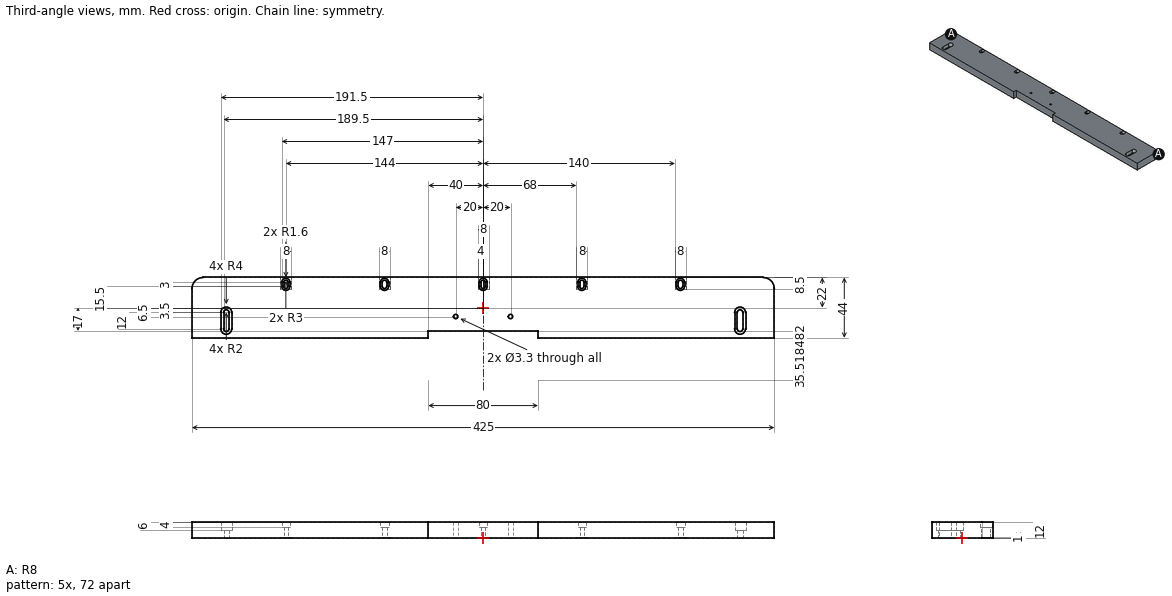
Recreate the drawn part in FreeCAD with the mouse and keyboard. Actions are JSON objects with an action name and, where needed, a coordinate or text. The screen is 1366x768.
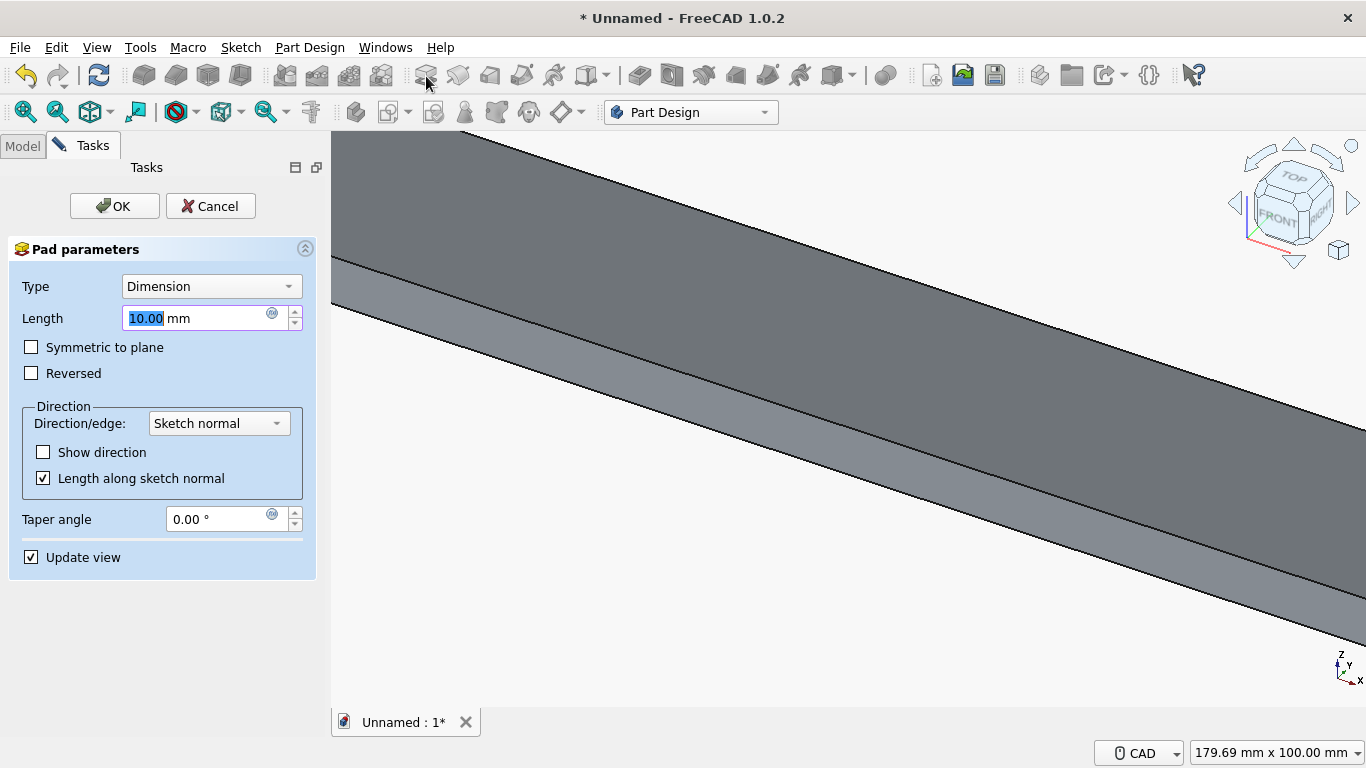
{"action": "type", "text": "12"}
{"action": "key", "text": "Tab"}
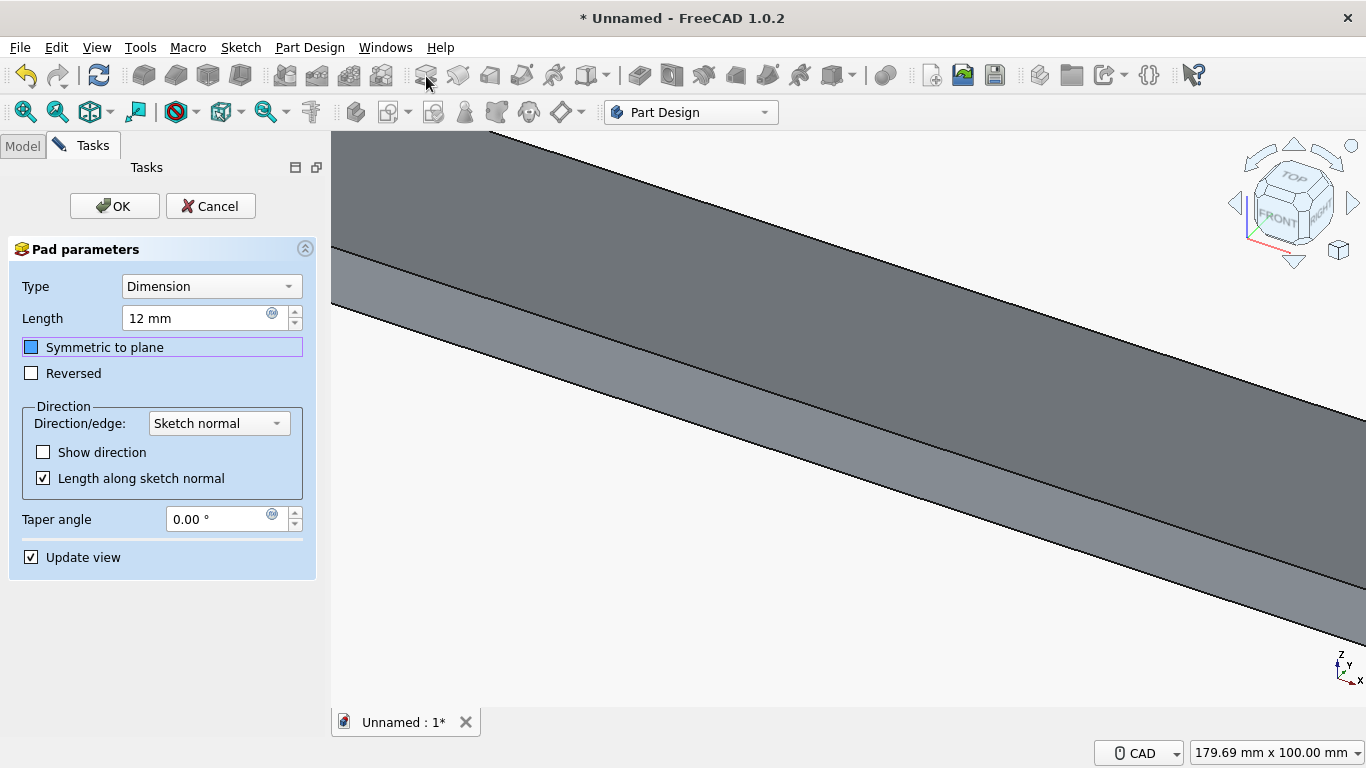
{"action": "left_click", "coordinate": [115, 206]}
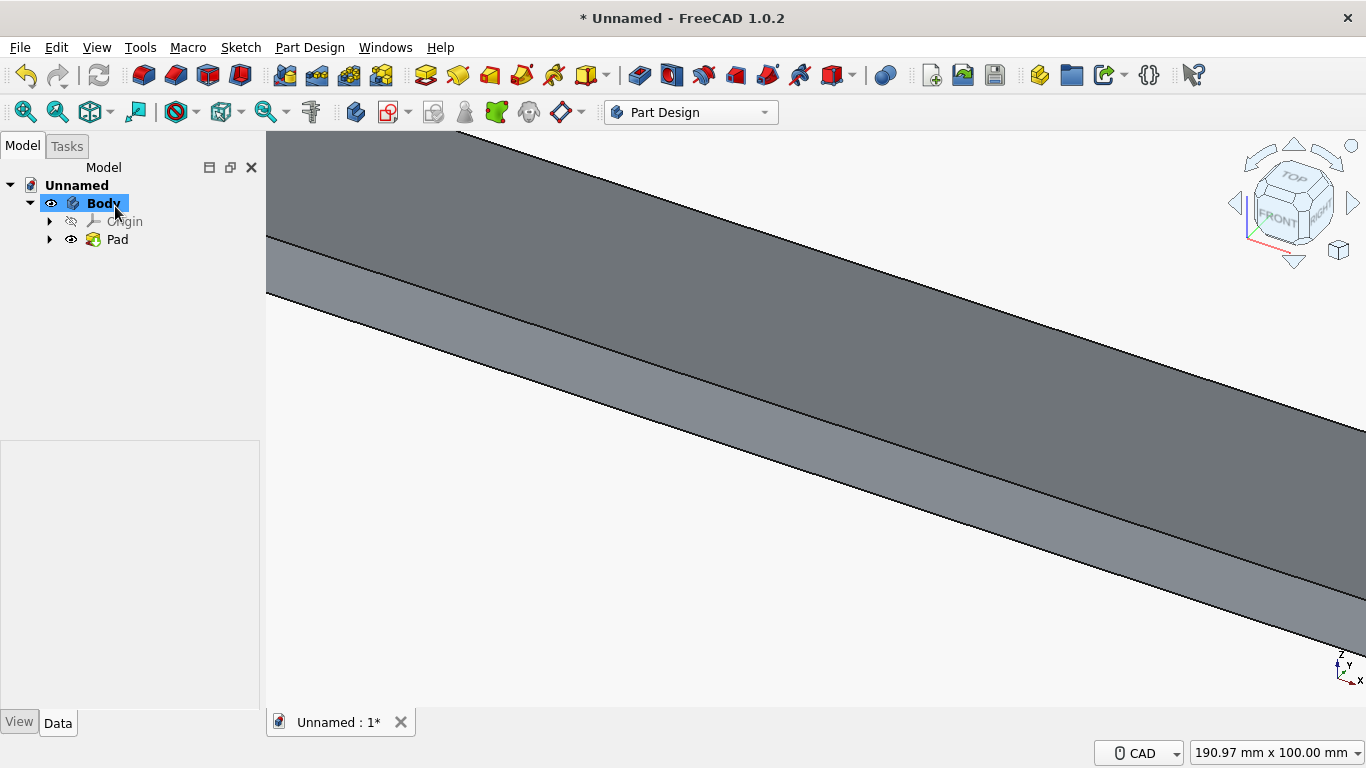
{"action": "left_click", "coordinate": [26, 112]}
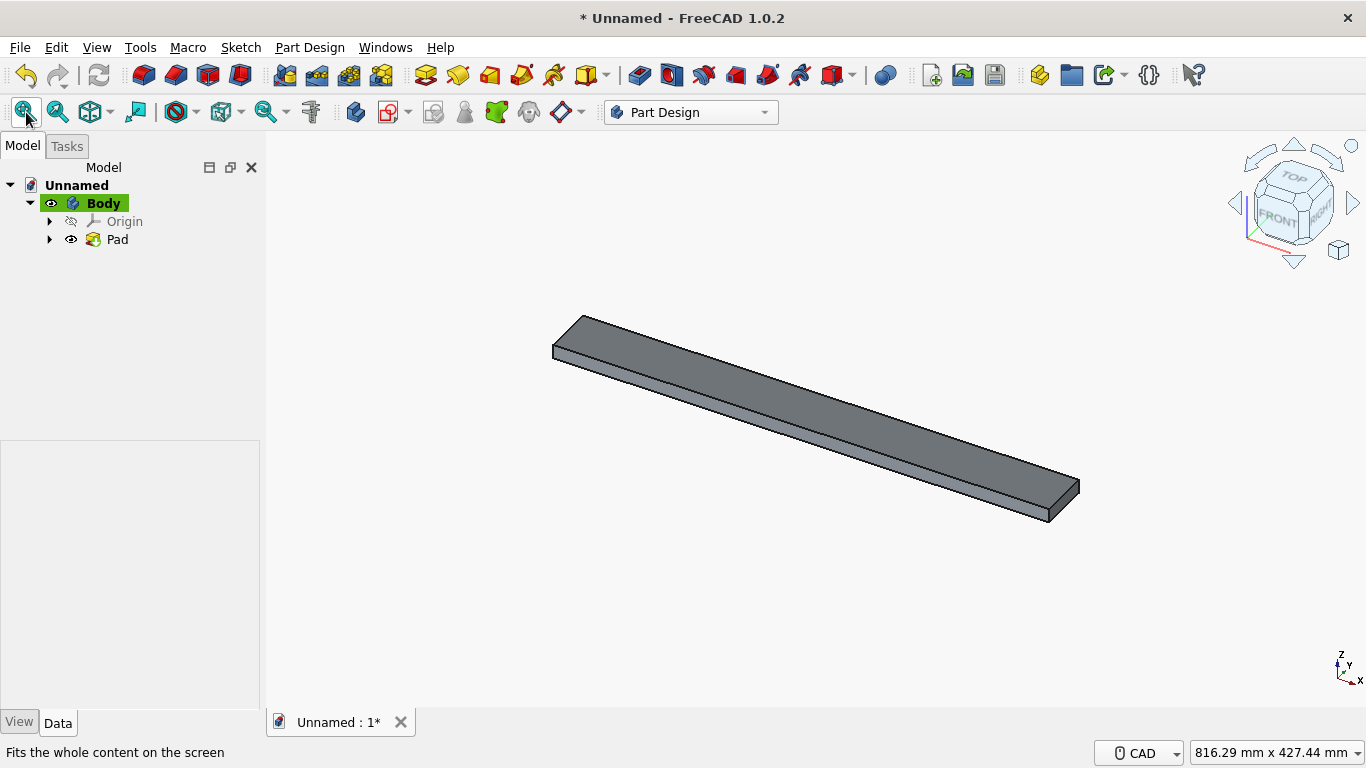
{"action": "scroll", "coordinate": [583, 321], "scroll_direction": "up", "scroll_amount": 5}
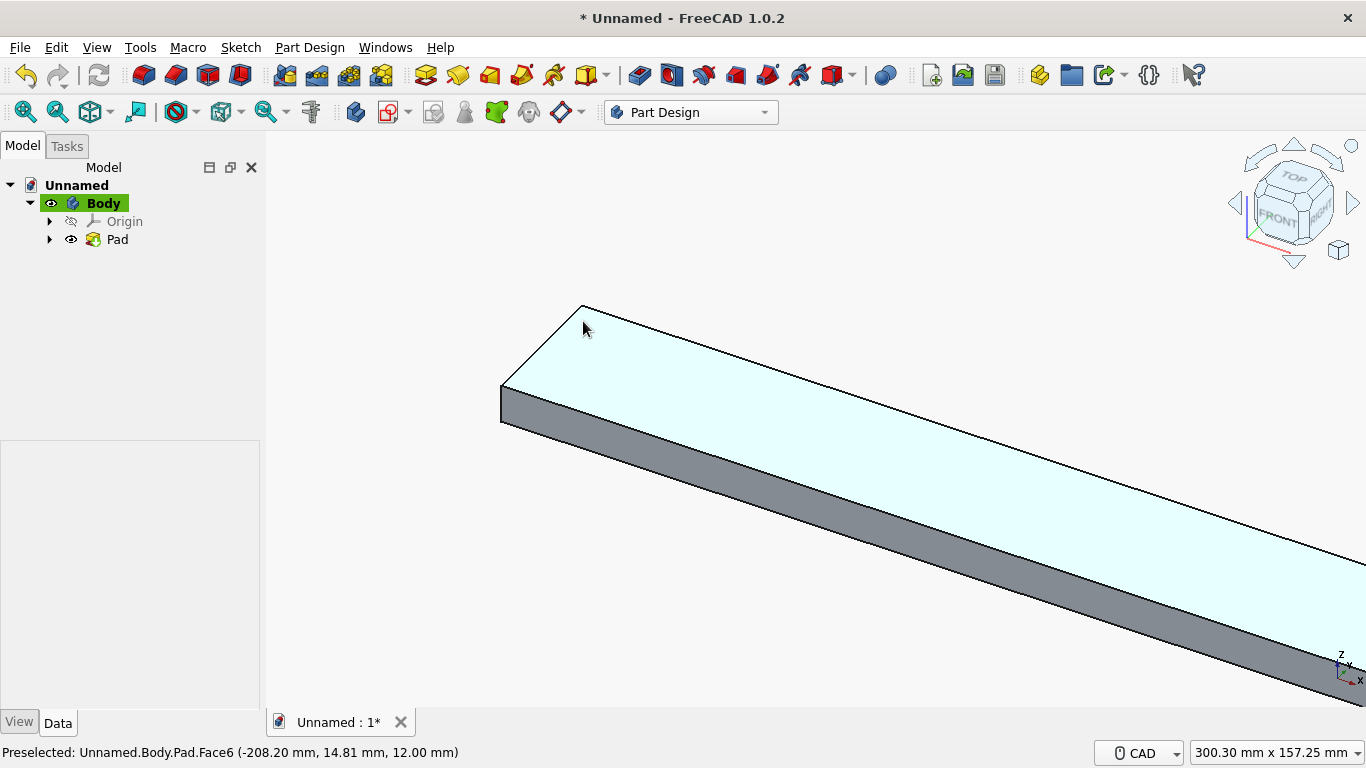
{"action": "key", "text": "v f"}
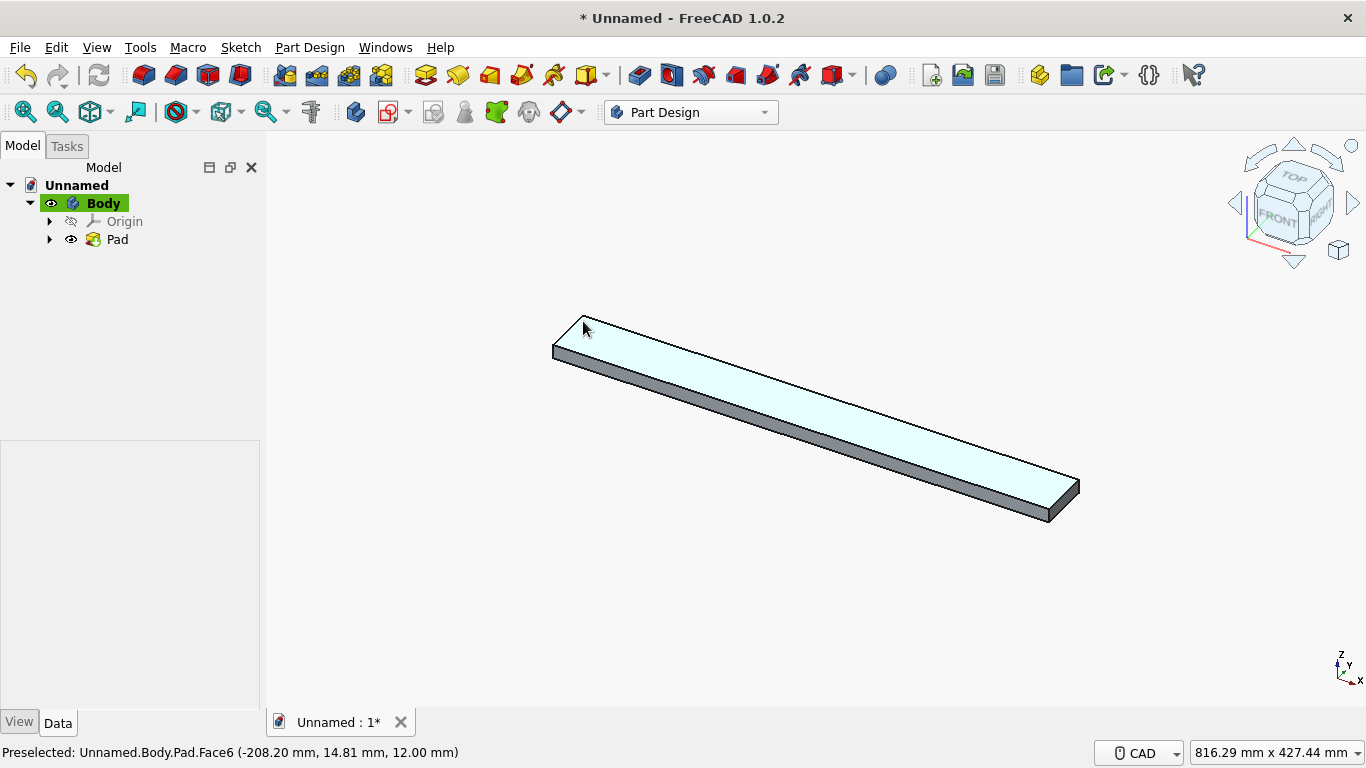
{"action": "key", "text": "0"}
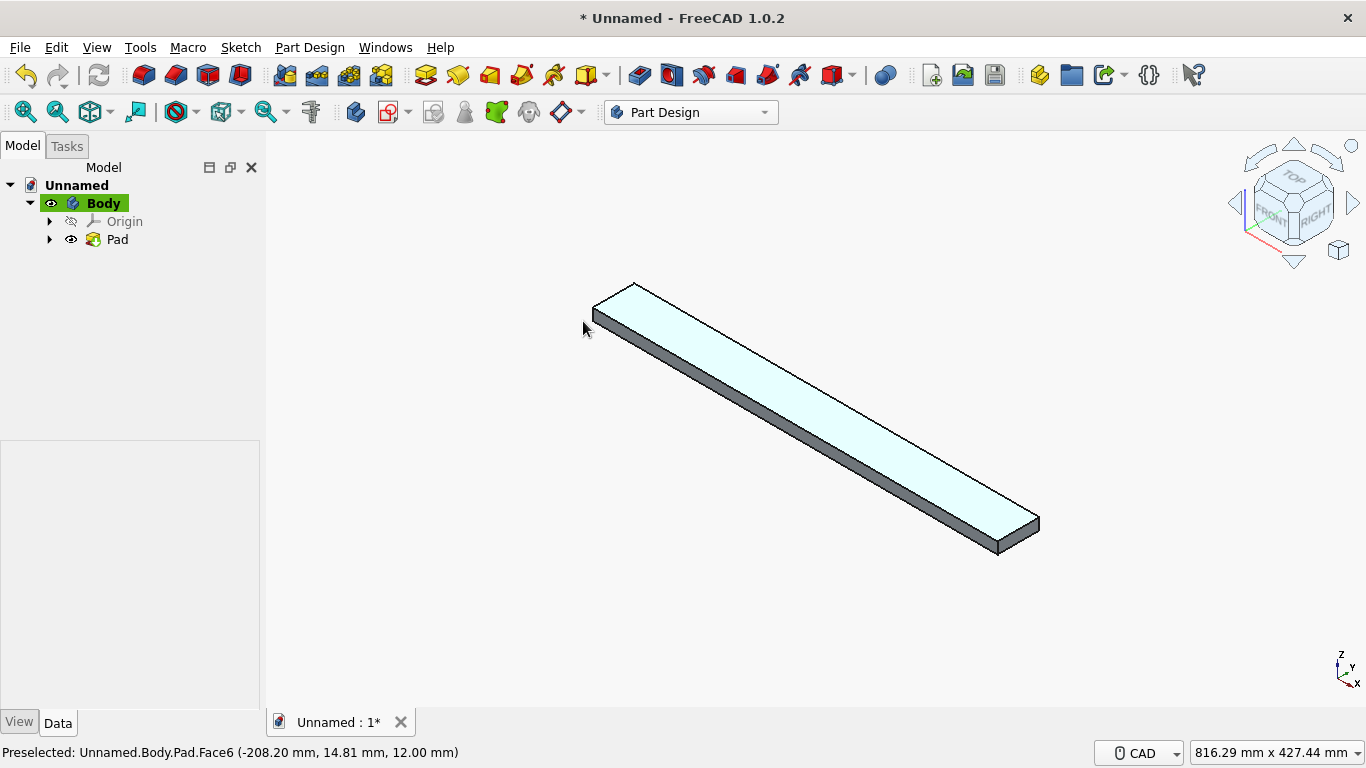
{"action": "scroll", "coordinate": [634, 289], "scroll_direction": "up", "scroll_amount": 5}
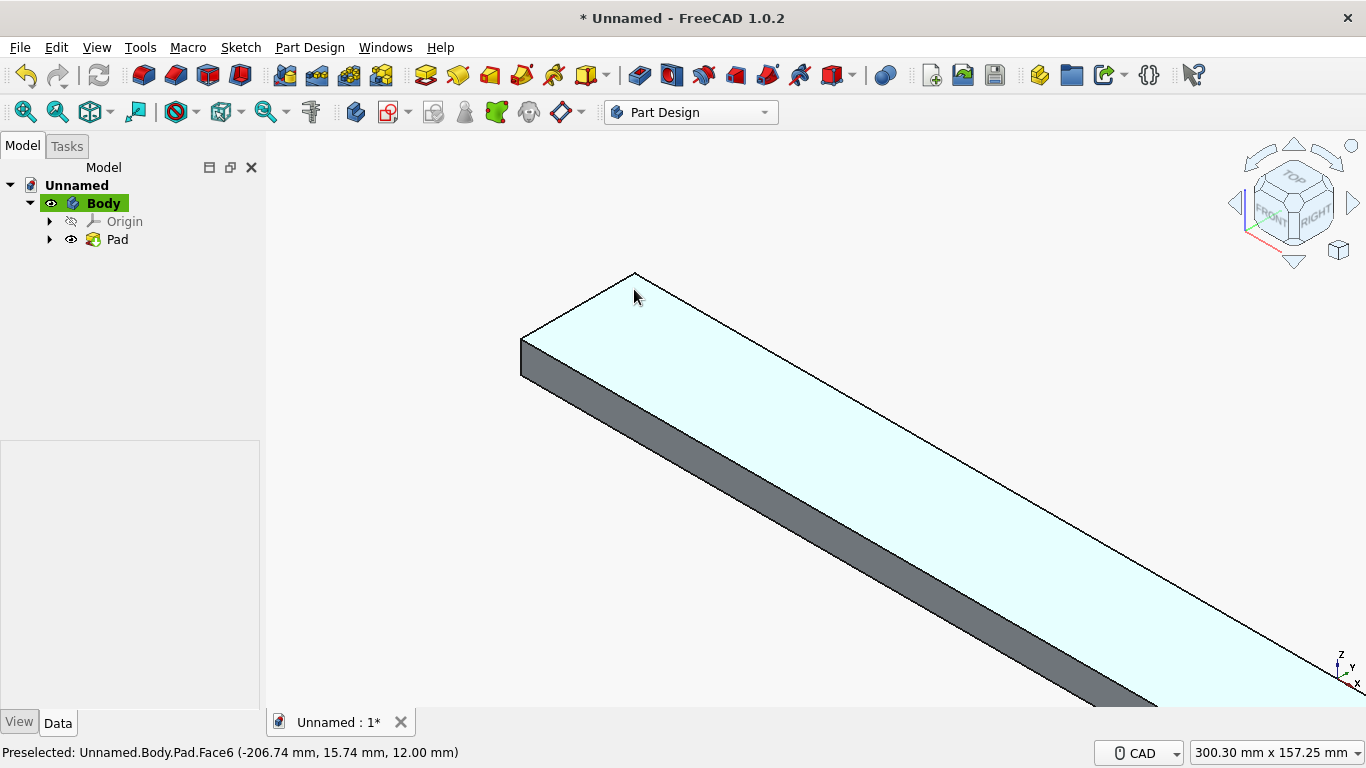
{"action": "left_click", "coordinate": [26, 112]}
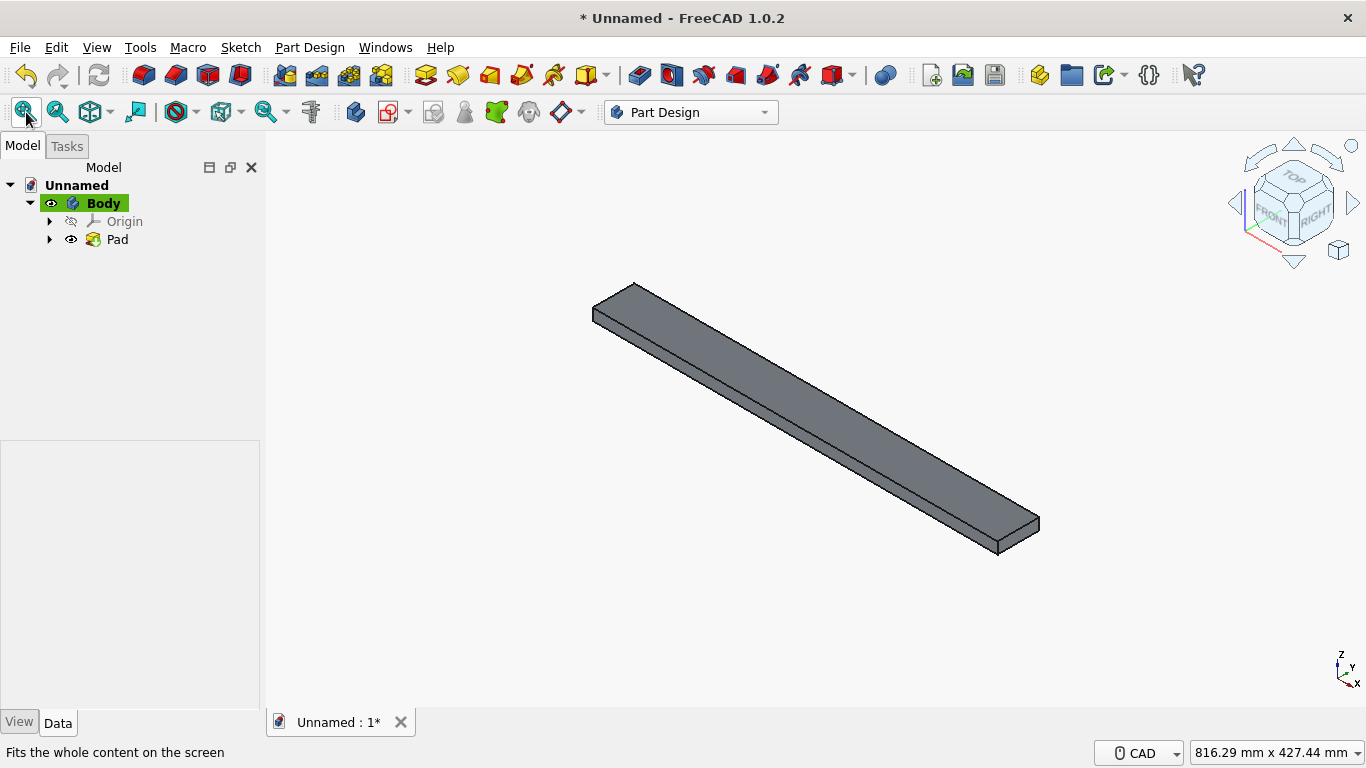
{"action": "key", "text": "2"}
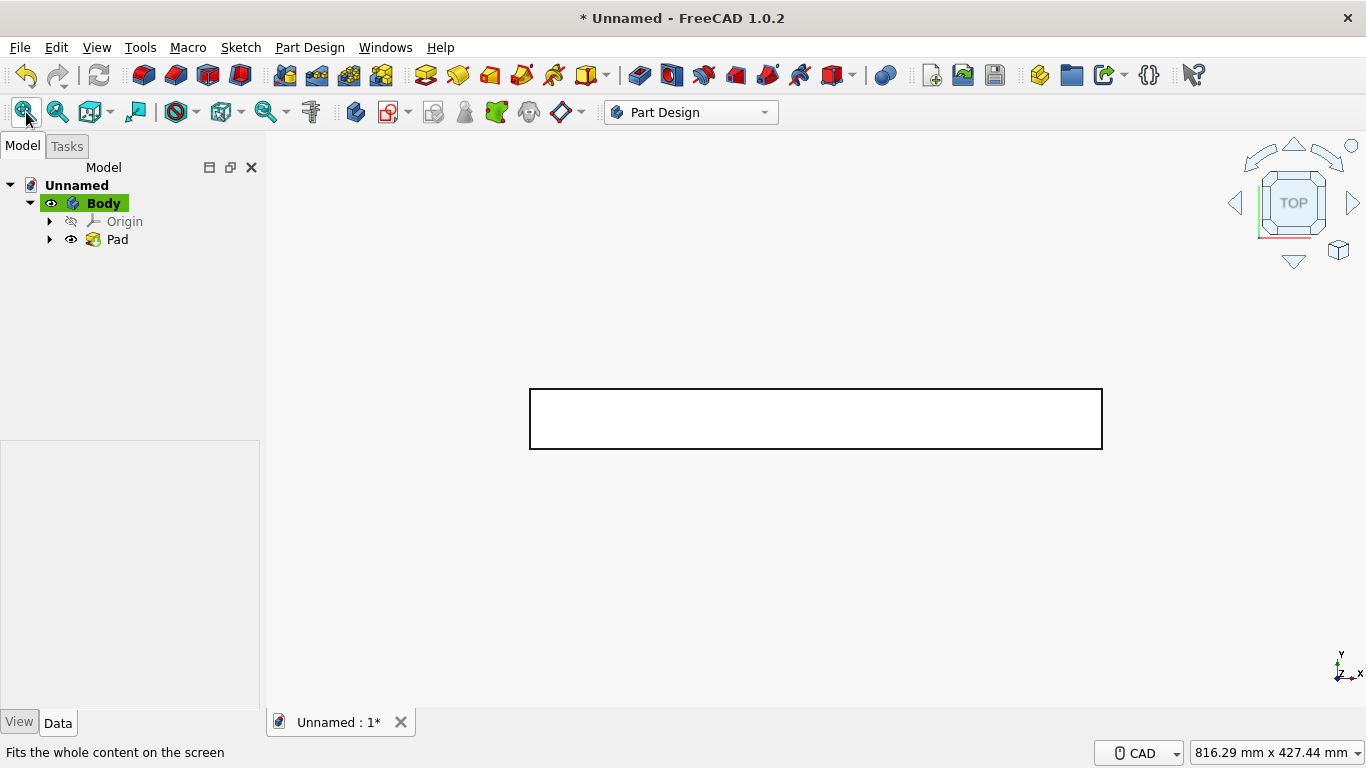
{"action": "scroll", "coordinate": [530, 388], "scroll_direction": "up", "scroll_amount": 5}